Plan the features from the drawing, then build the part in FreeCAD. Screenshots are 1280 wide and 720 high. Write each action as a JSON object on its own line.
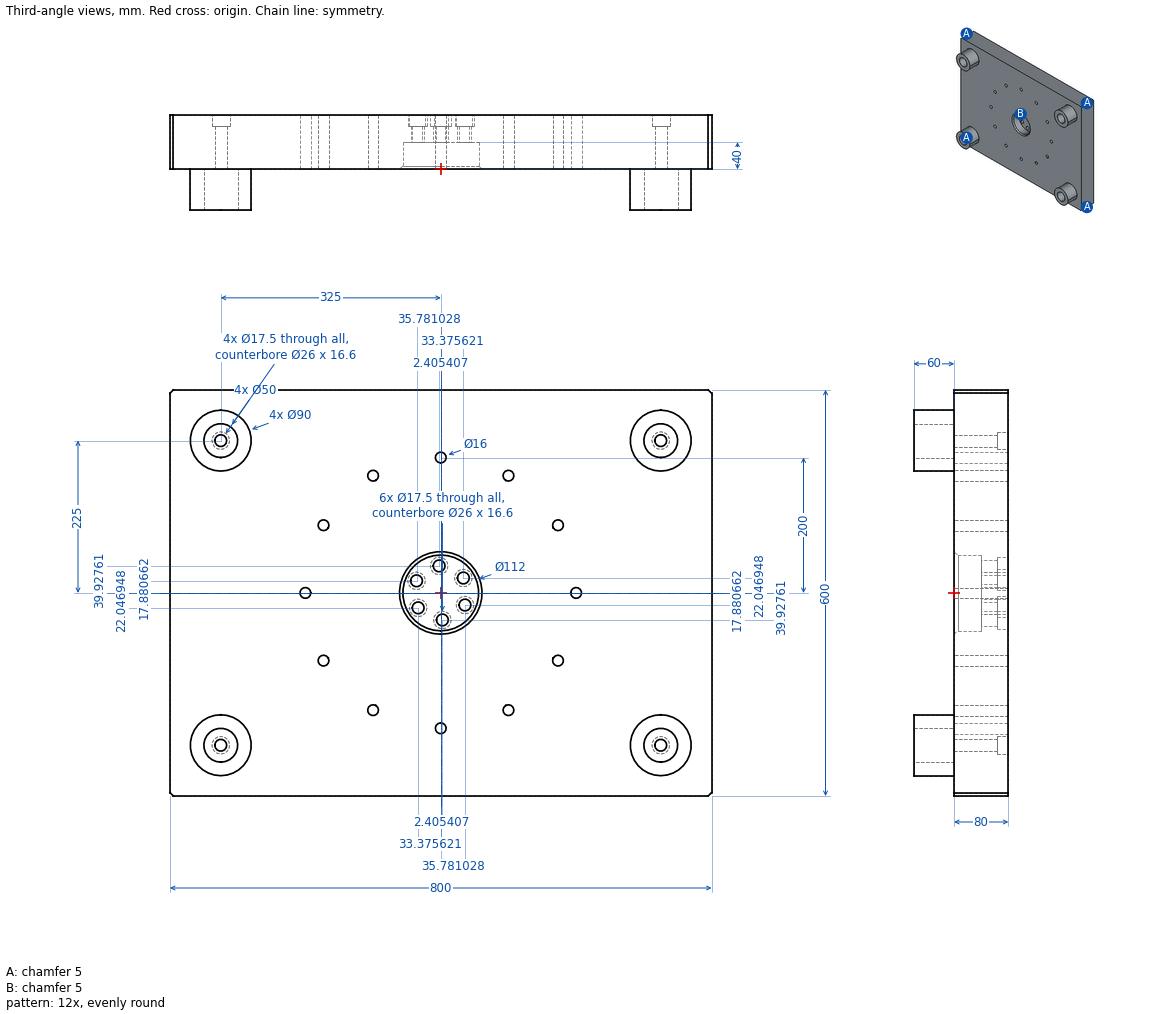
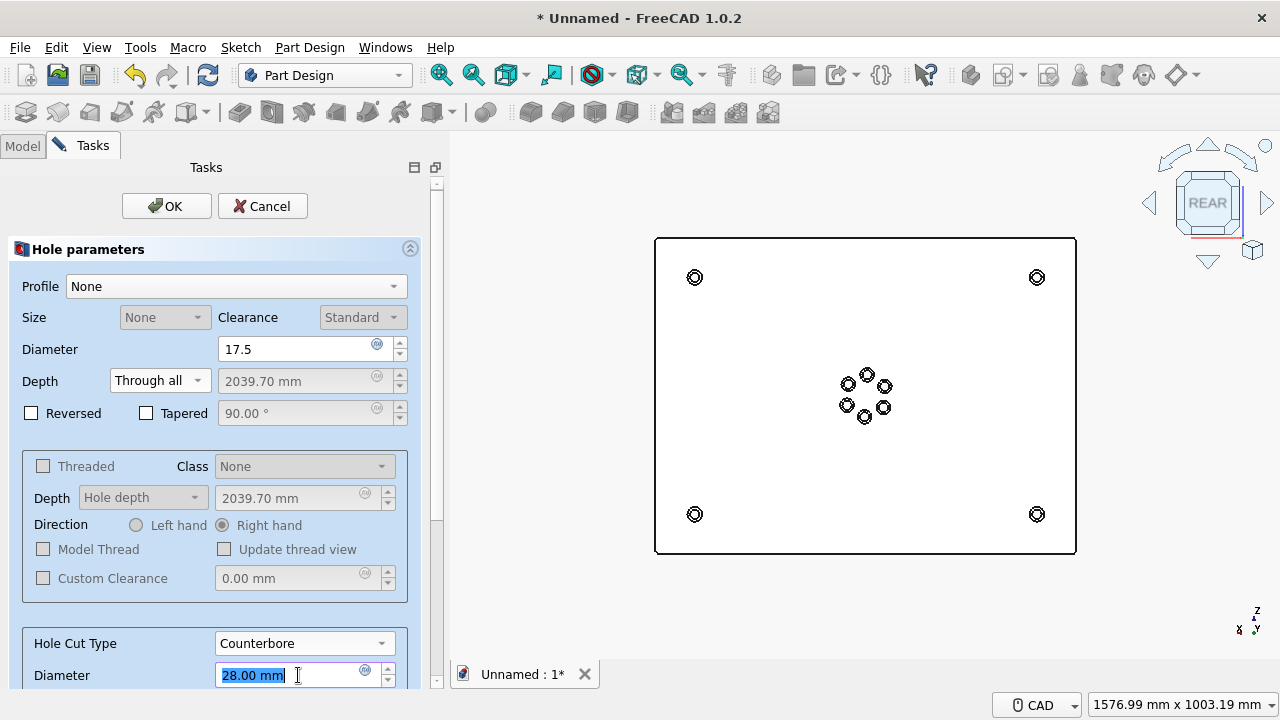
{"action": "type", "text": "26"}
{"action": "key", "text": "Tab"}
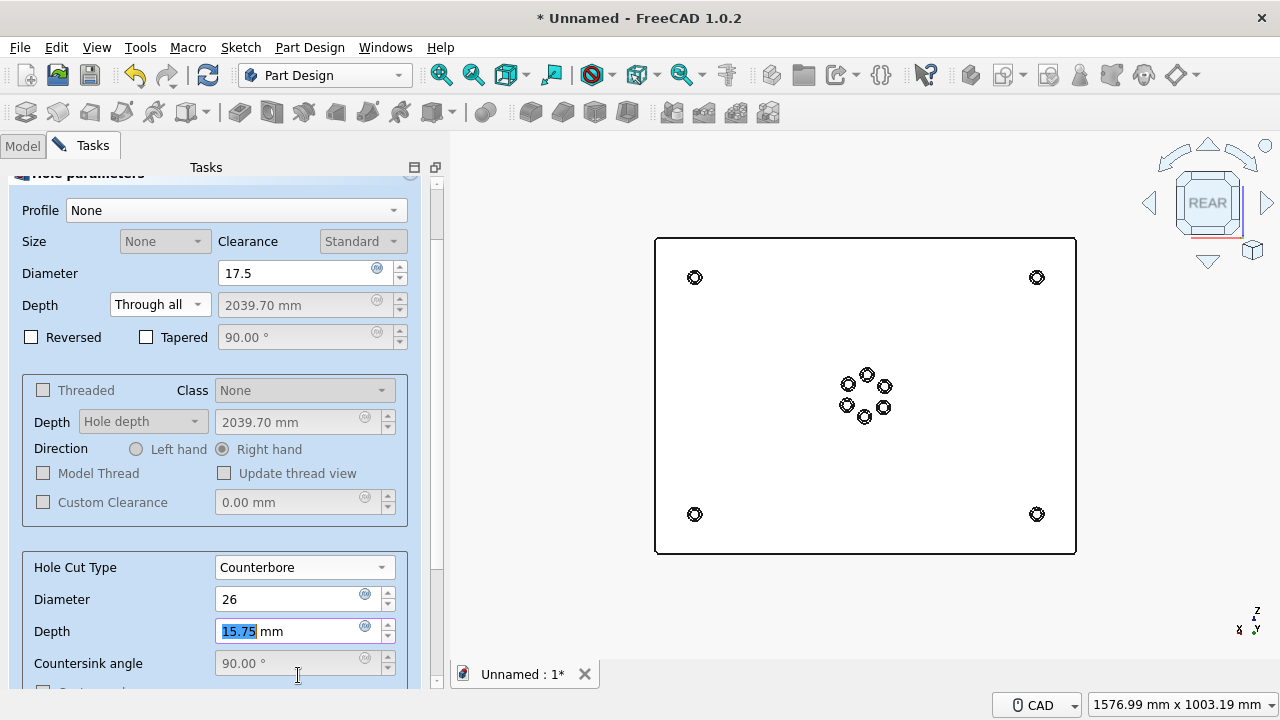
{"action": "type", "text": "16.6"}
{"action": "key", "text": "Tab"}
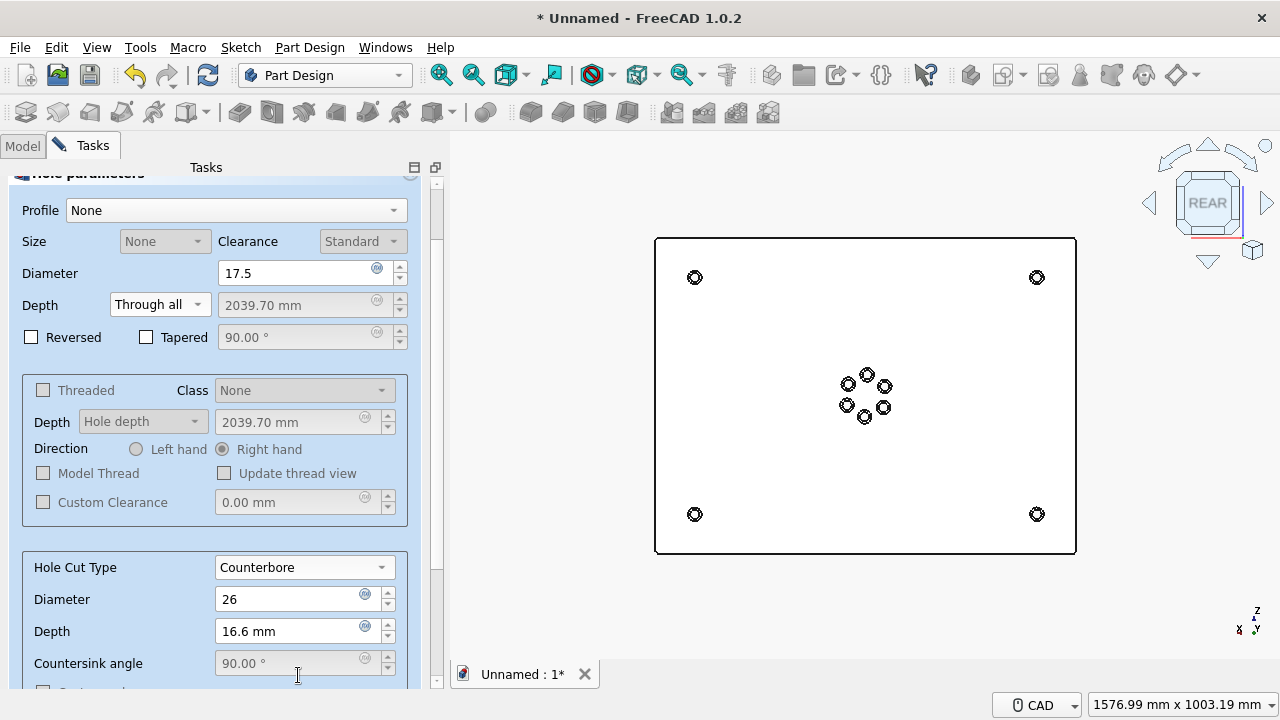
{"action": "scroll", "coordinate": [437, 432], "scroll_direction": "up", "scroll_amount": 3}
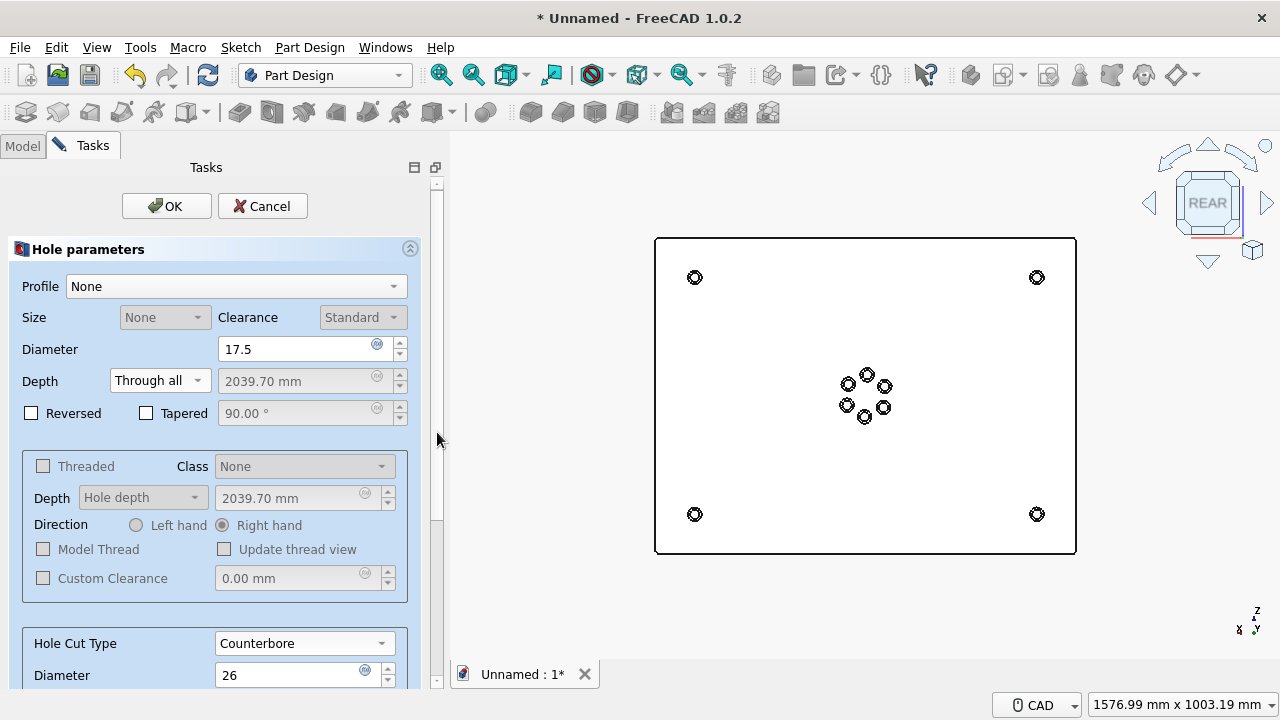
{"action": "left_click", "coordinate": [167, 206]}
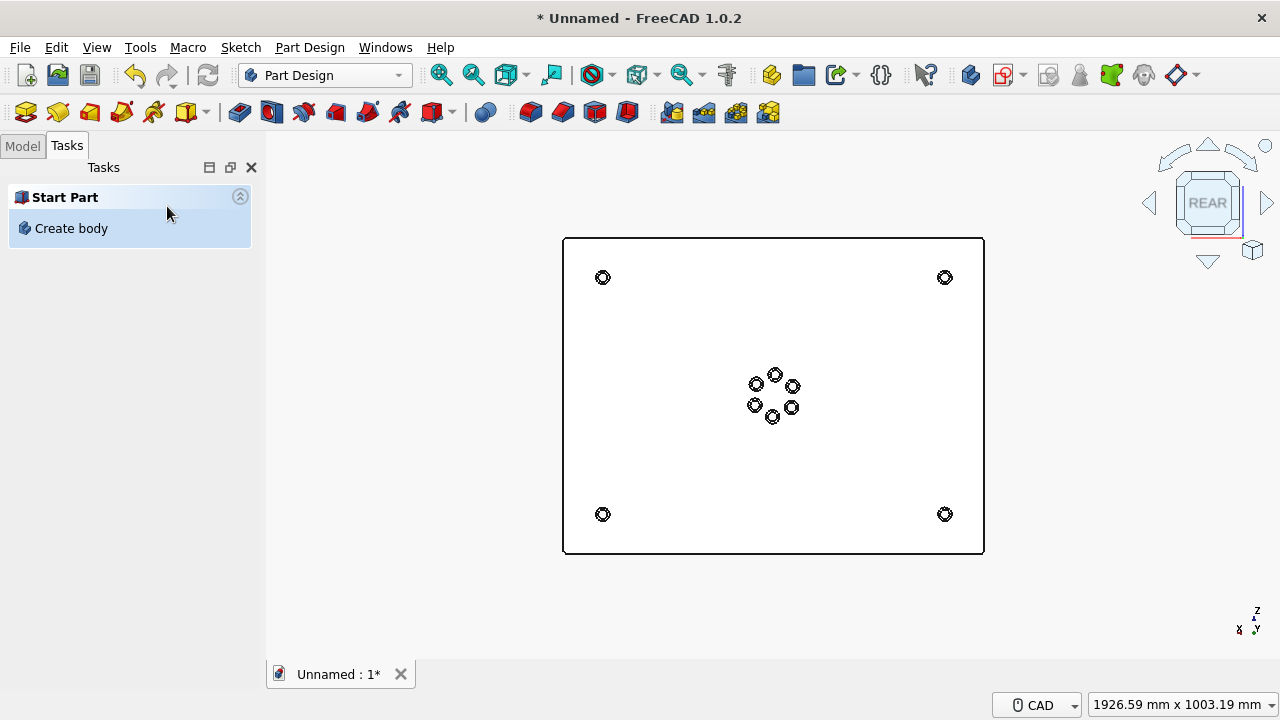
{"action": "key", "text": "0"}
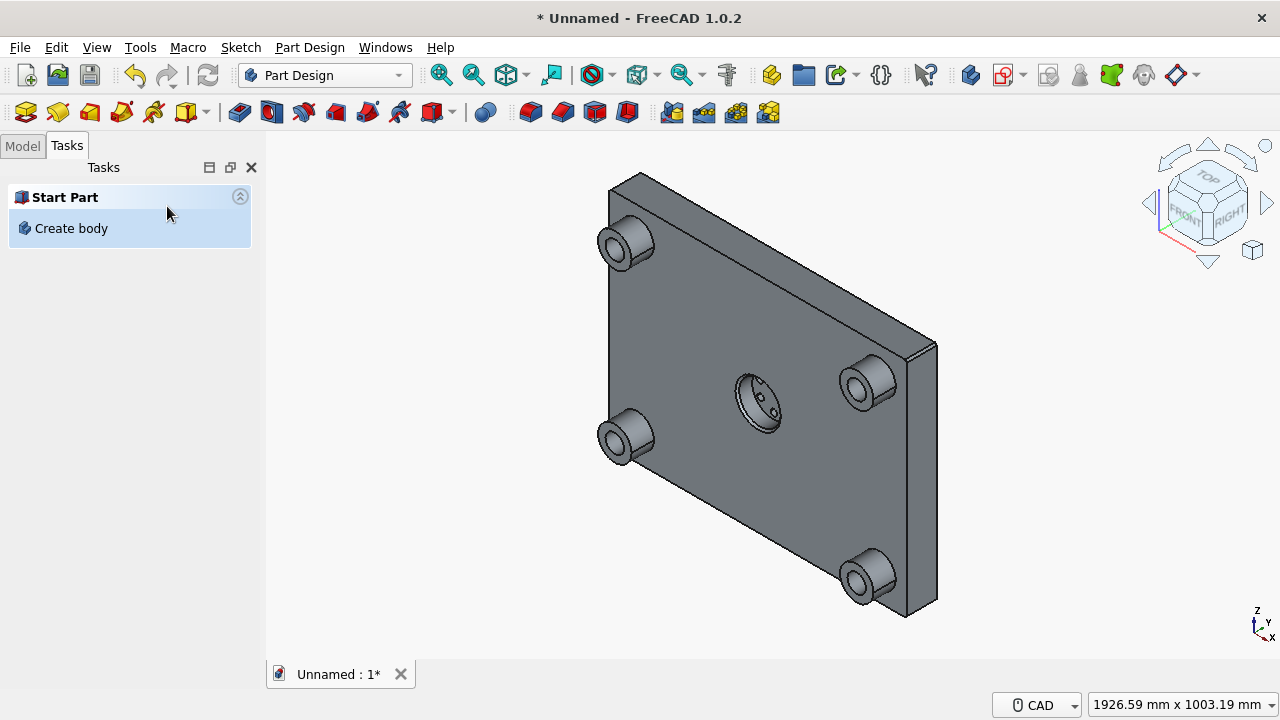
{"action": "left_click", "coordinate": [843, 452]}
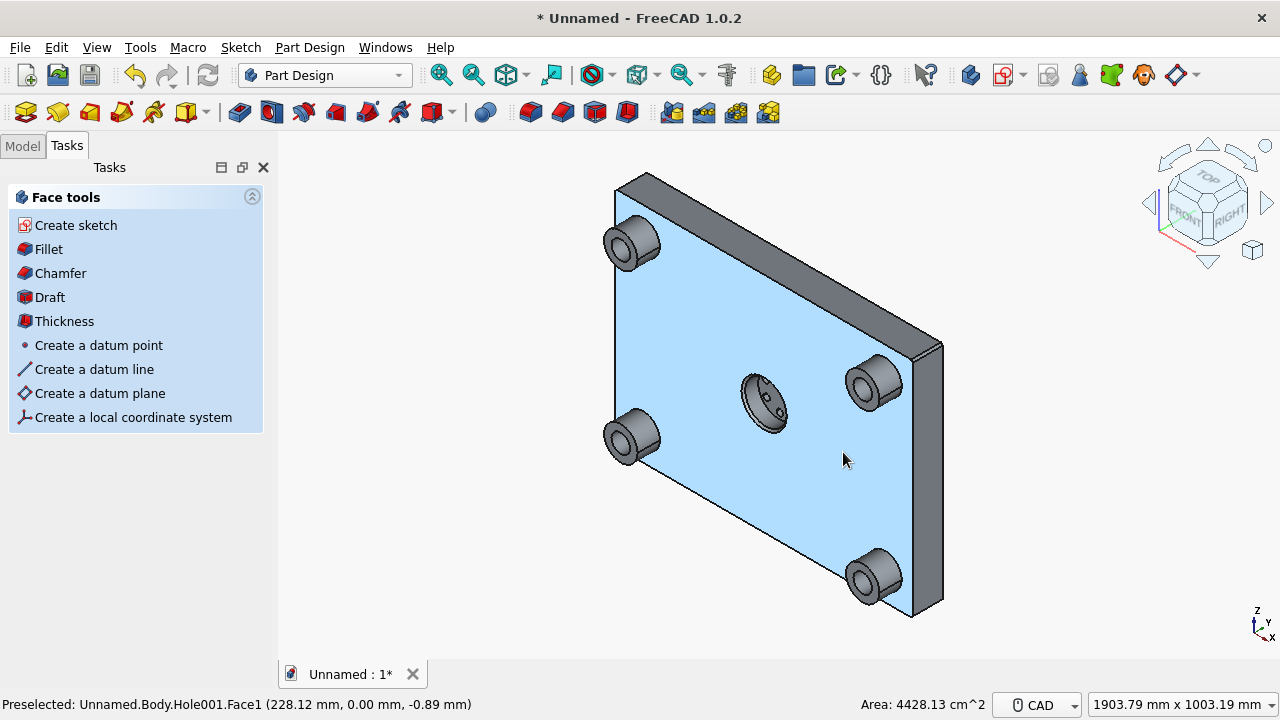
{"action": "left_click", "coordinate": [1004, 76]}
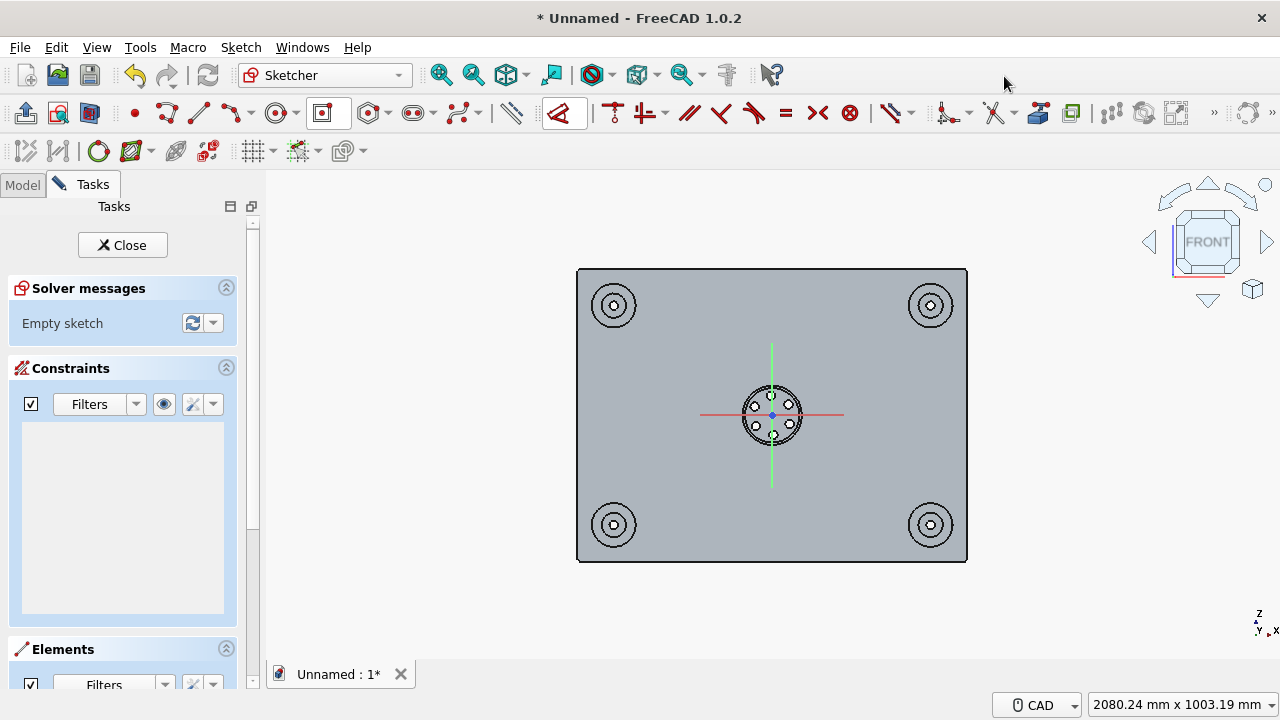
{"action": "key", "text": "q s"}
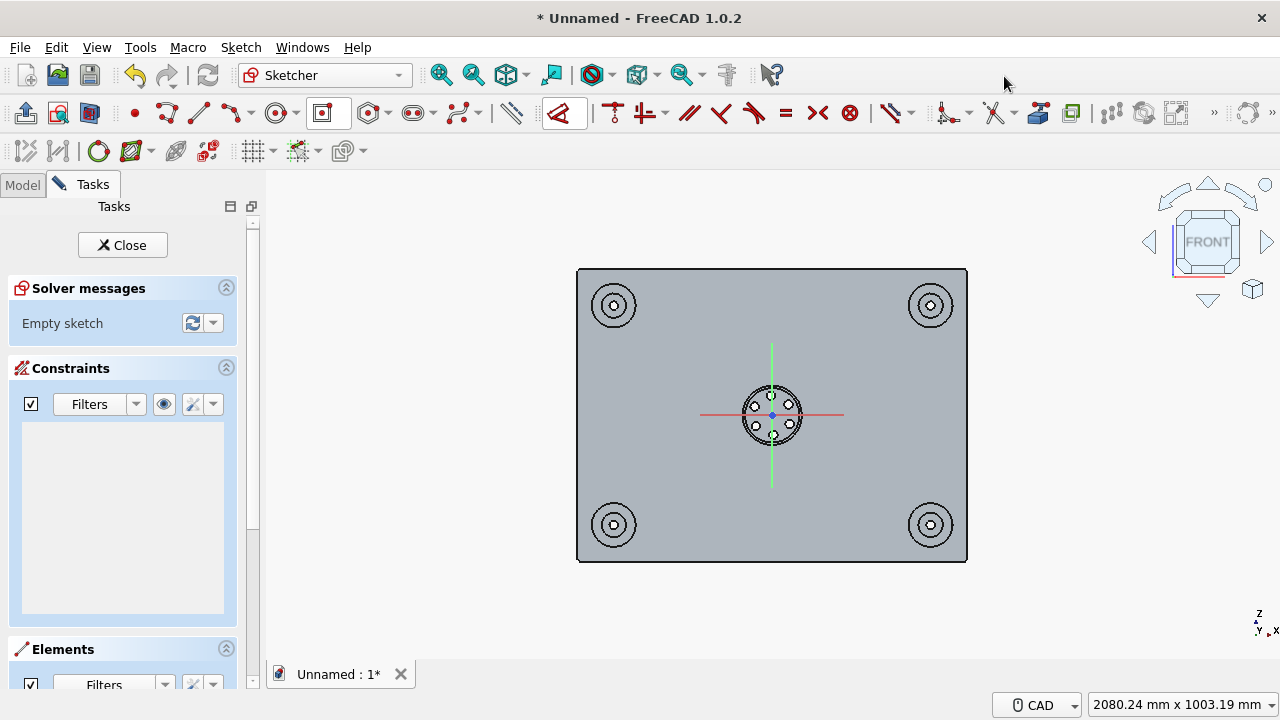
{"action": "scroll", "coordinate": [776, 313], "scroll_direction": "up", "scroll_amount": 15}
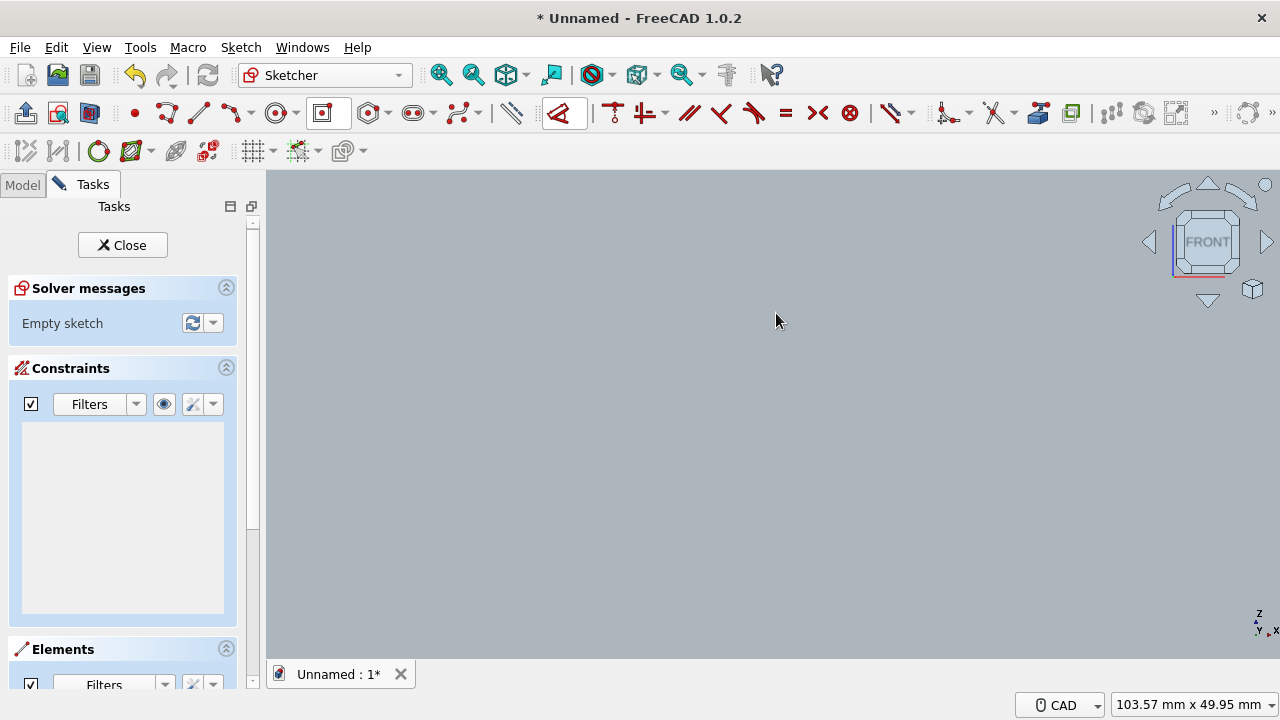
{"action": "scroll", "coordinate": [672, 392], "scroll_direction": "up", "scroll_amount": 3}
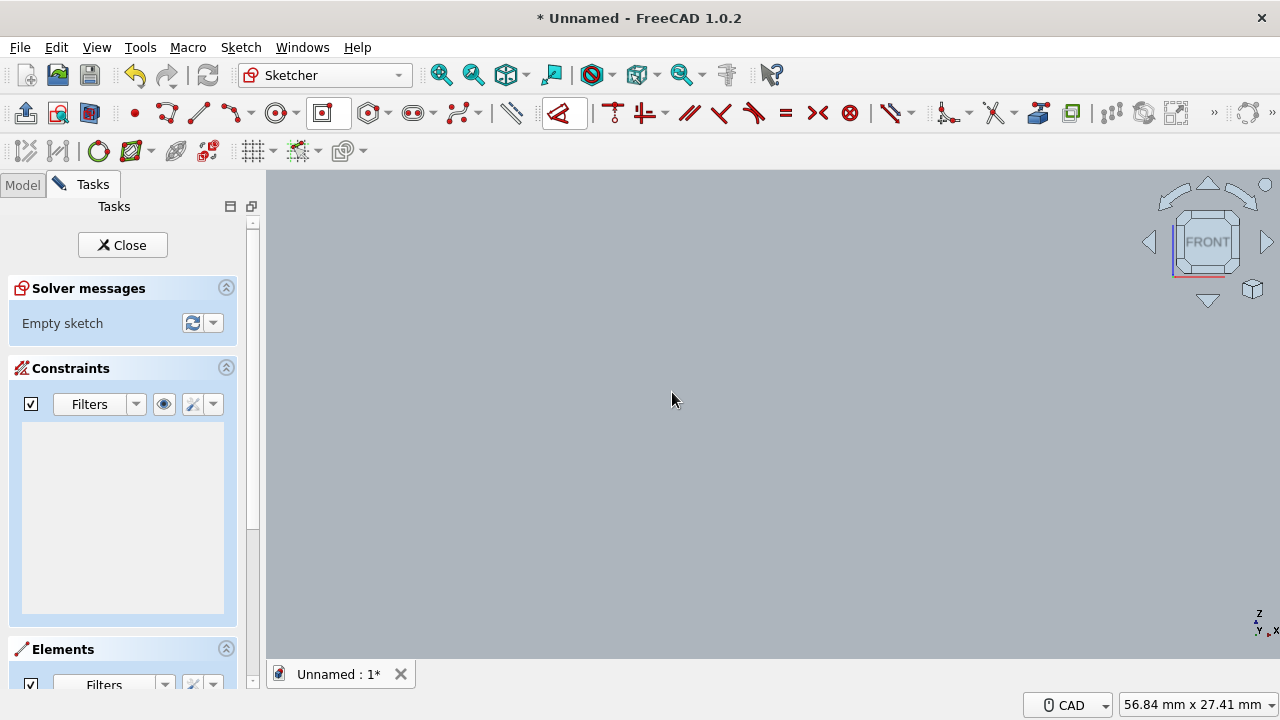
{"action": "key", "text": "g c"}